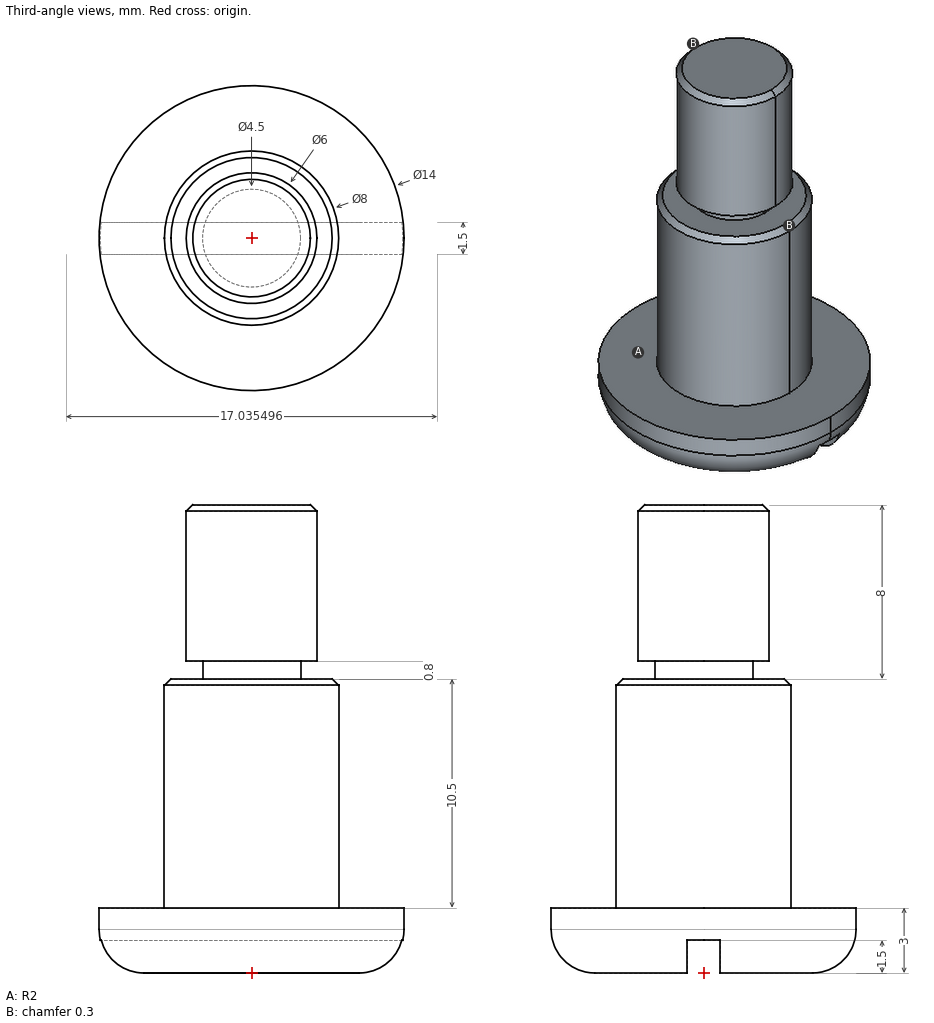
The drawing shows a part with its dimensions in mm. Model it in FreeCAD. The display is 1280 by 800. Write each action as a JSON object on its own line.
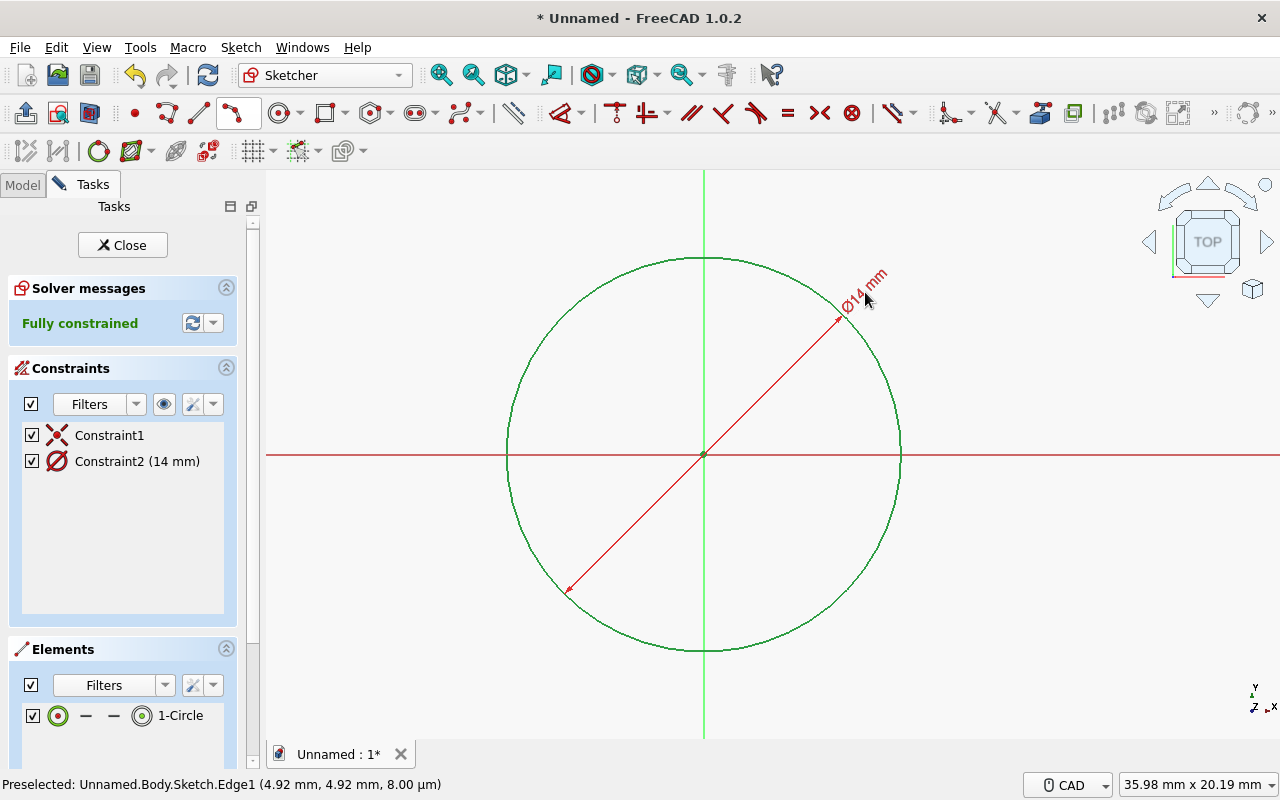
{"action": "left_click", "coordinate": [123, 245]}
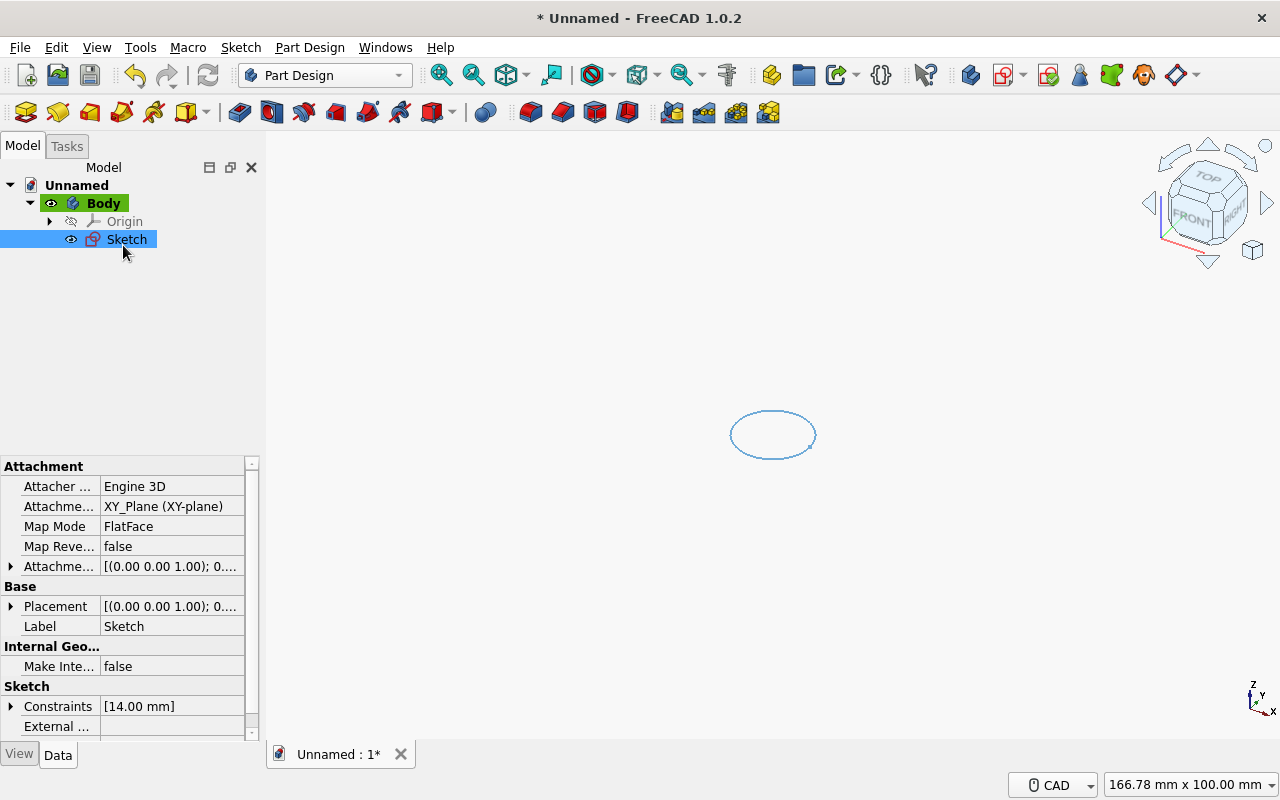
{"action": "left_click", "coordinate": [26, 112]}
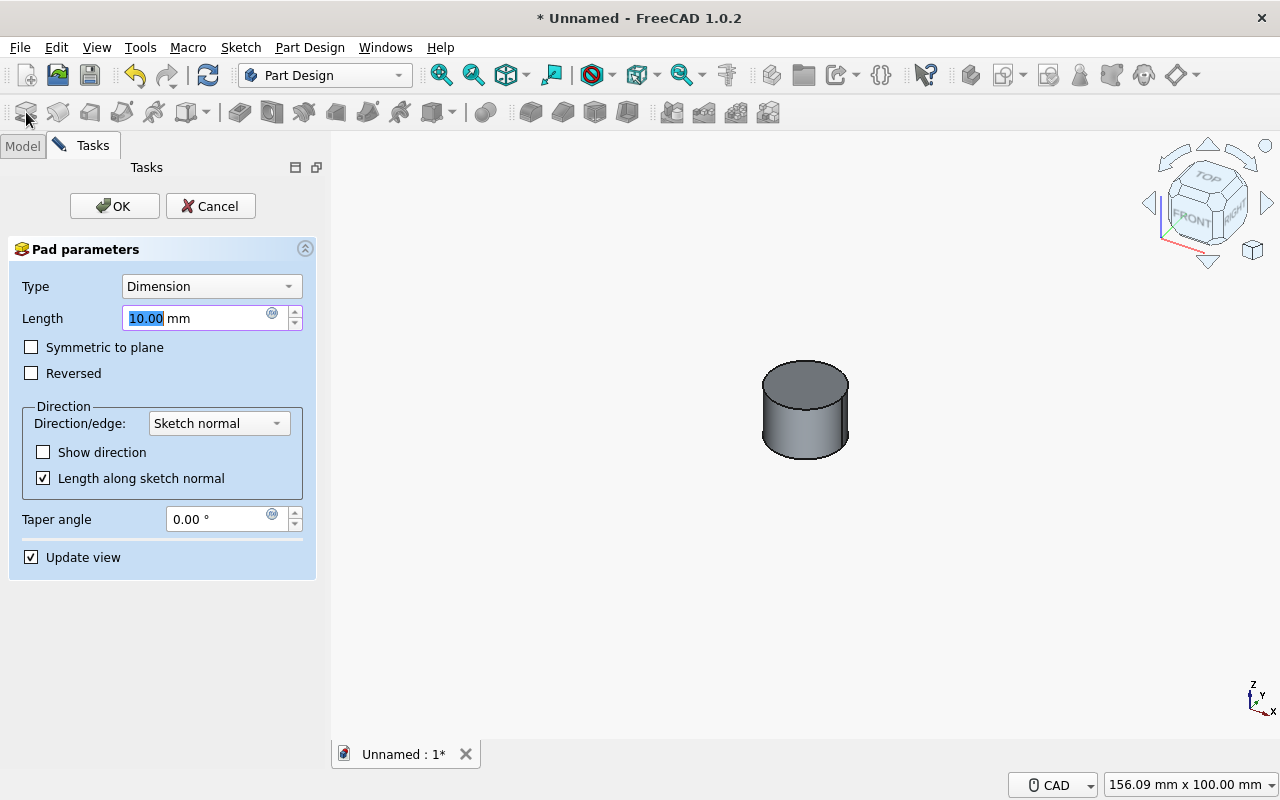
{"action": "type", "text": "3"}
{"action": "key", "text": "Tab"}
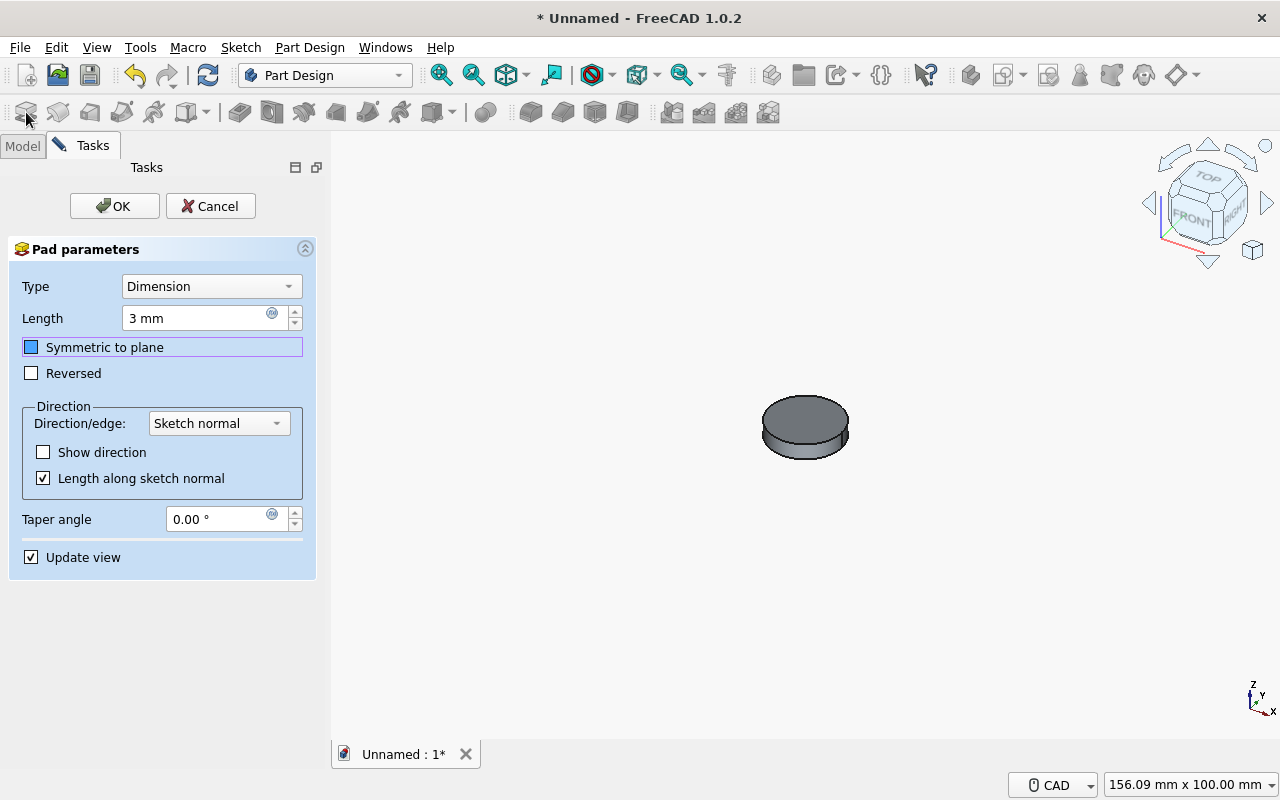
{"action": "left_click", "coordinate": [115, 206]}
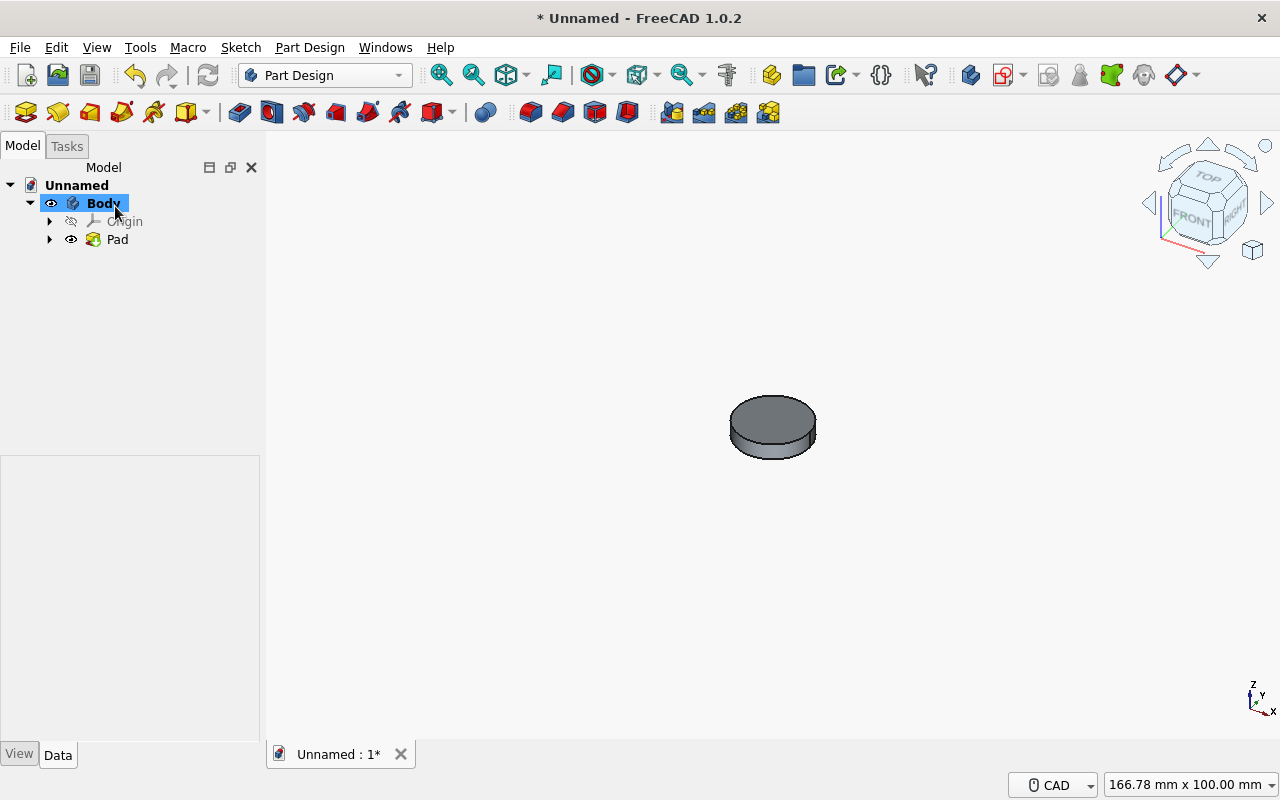
{"action": "left_click", "coordinate": [442, 76]}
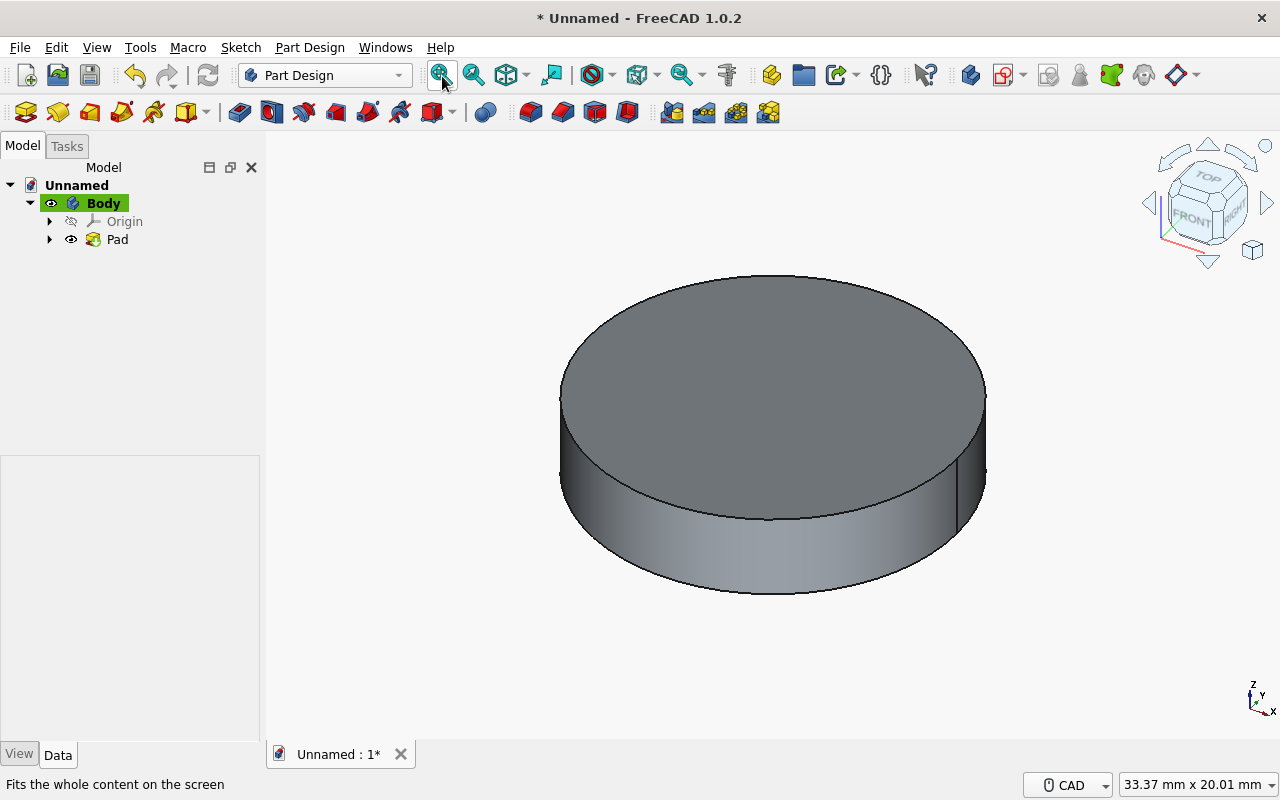
{"action": "left_click", "coordinate": [773, 397]}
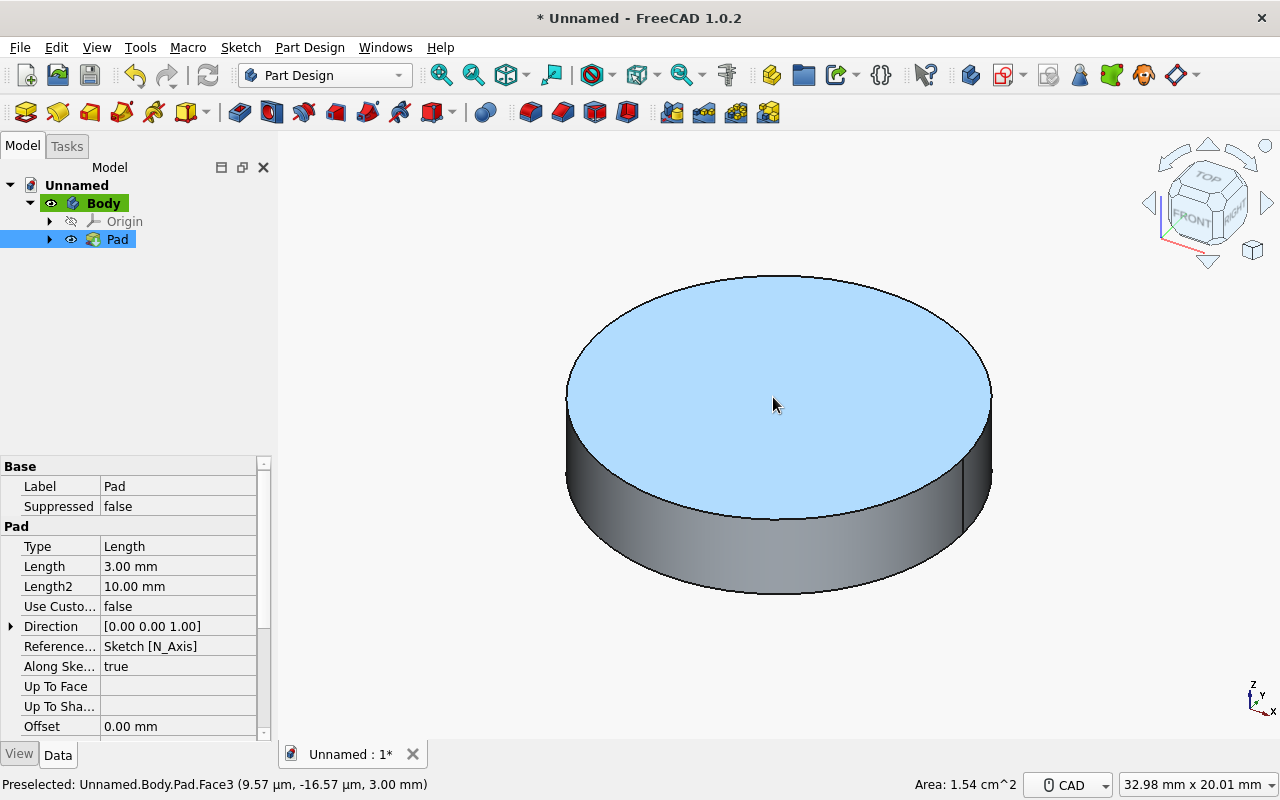
{"action": "left_click", "coordinate": [1004, 76]}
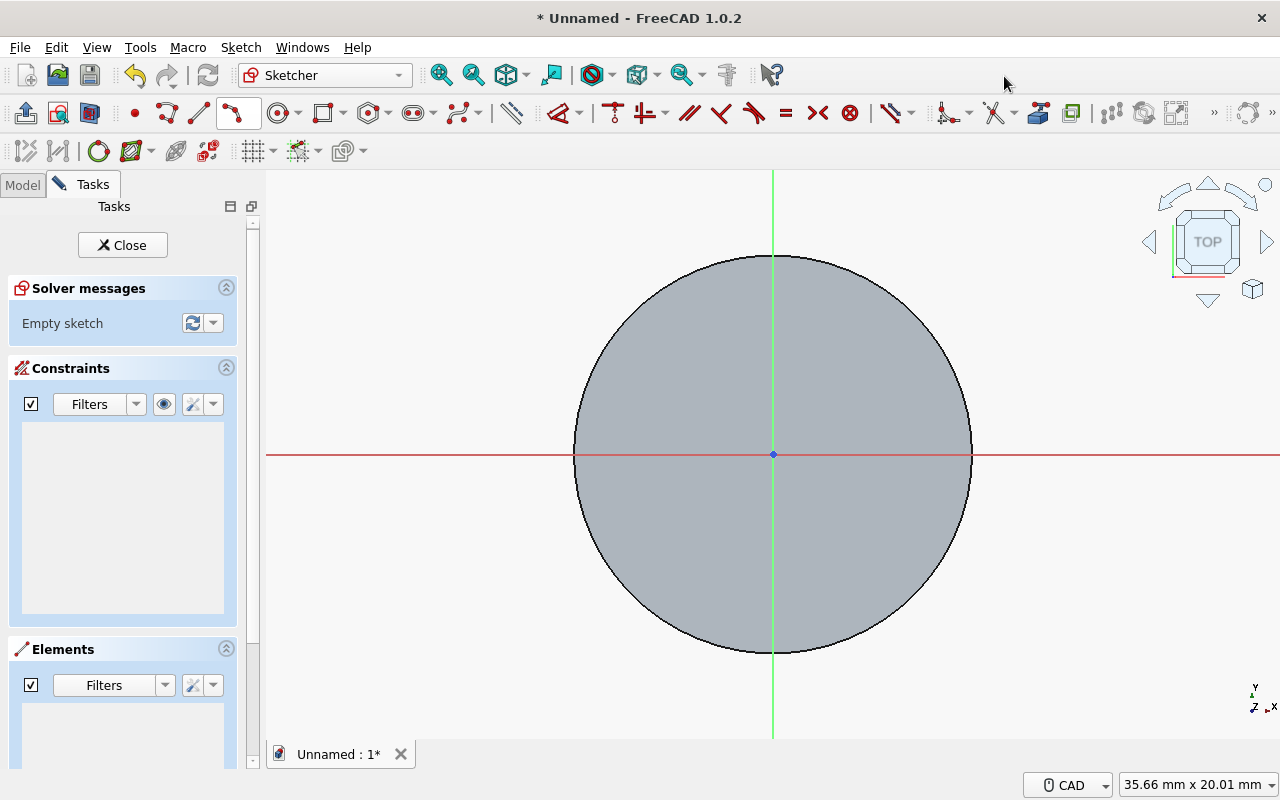
{"action": "scroll", "coordinate": [912, 455], "scroll_direction": "up", "scroll_amount": 2}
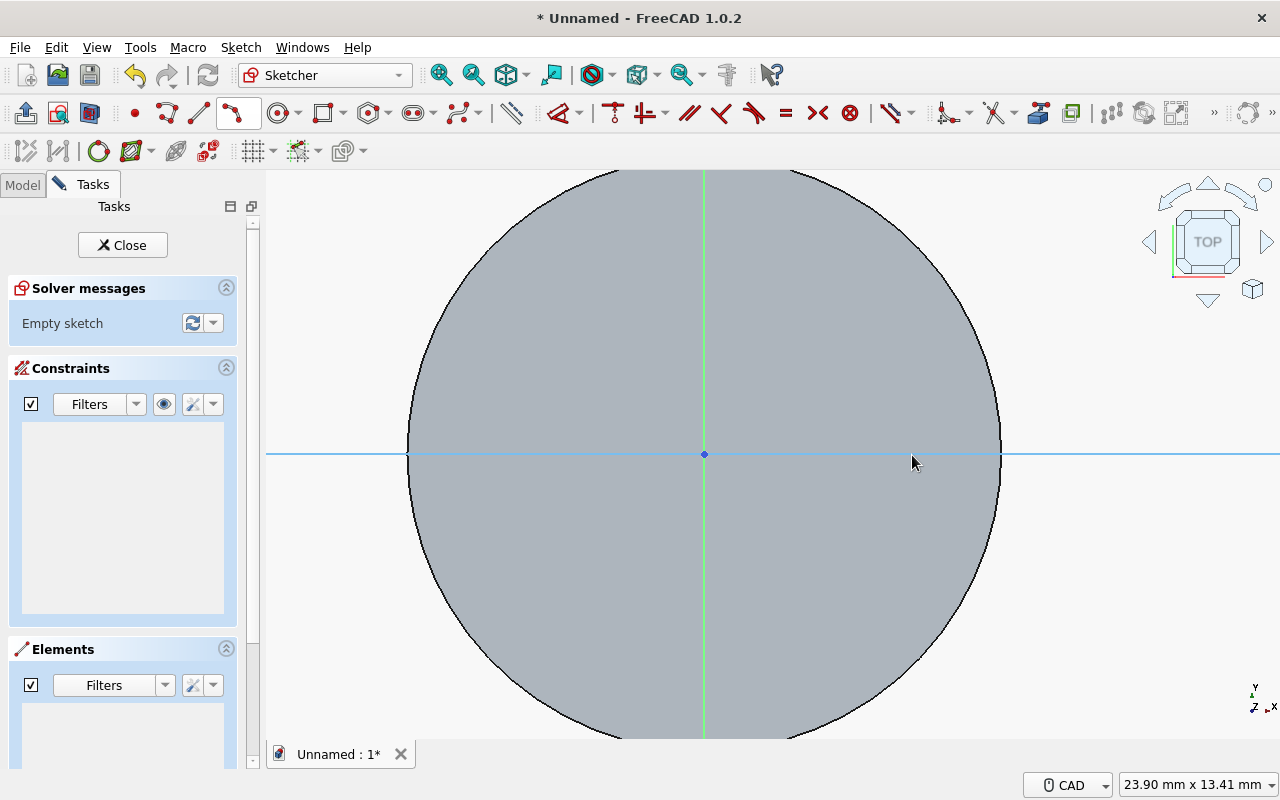
{"action": "left_click", "coordinate": [278, 114]}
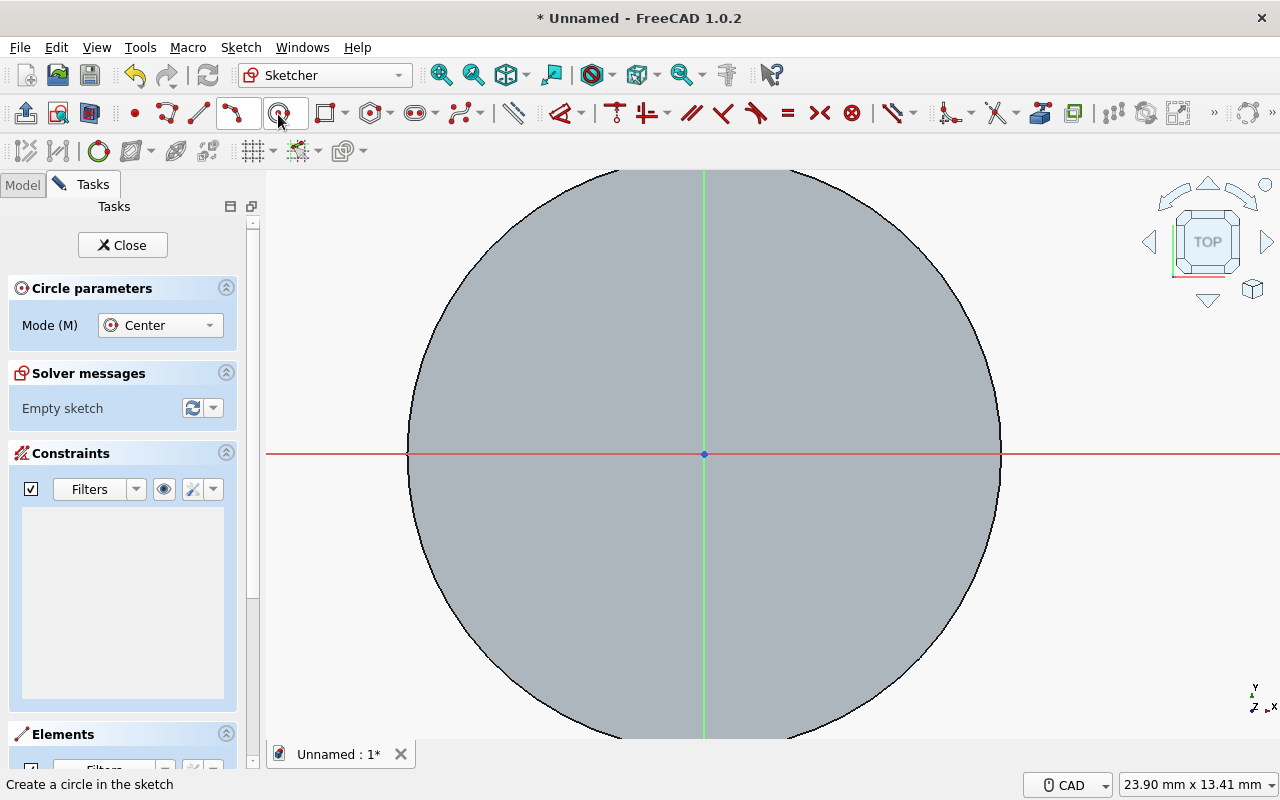
{"action": "left_click", "coordinate": [704, 454]}
{"action": "left_click", "coordinate": [824, 334]}
{"action": "key", "text": "Escape"}